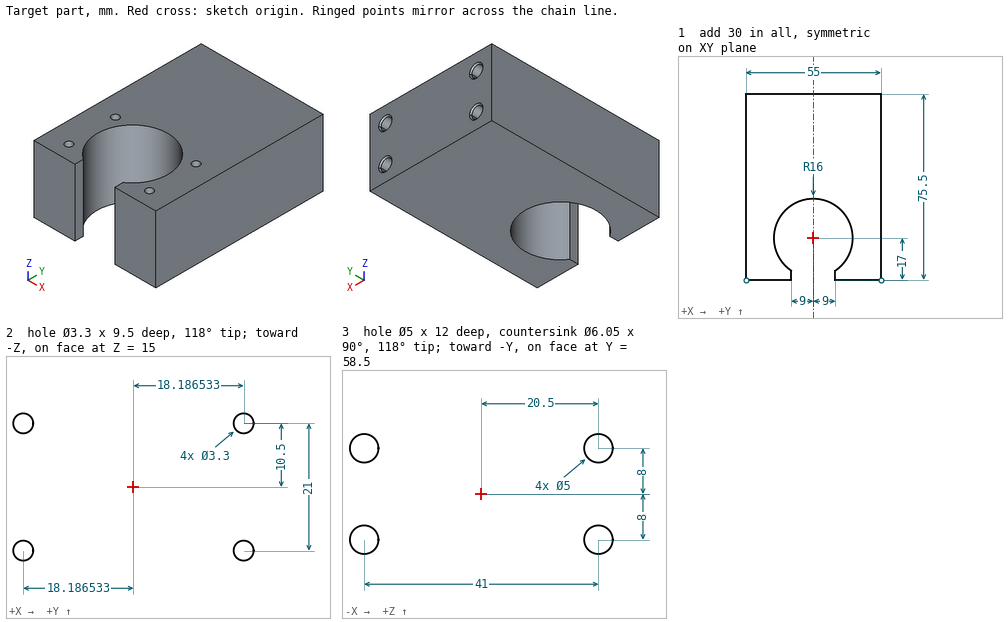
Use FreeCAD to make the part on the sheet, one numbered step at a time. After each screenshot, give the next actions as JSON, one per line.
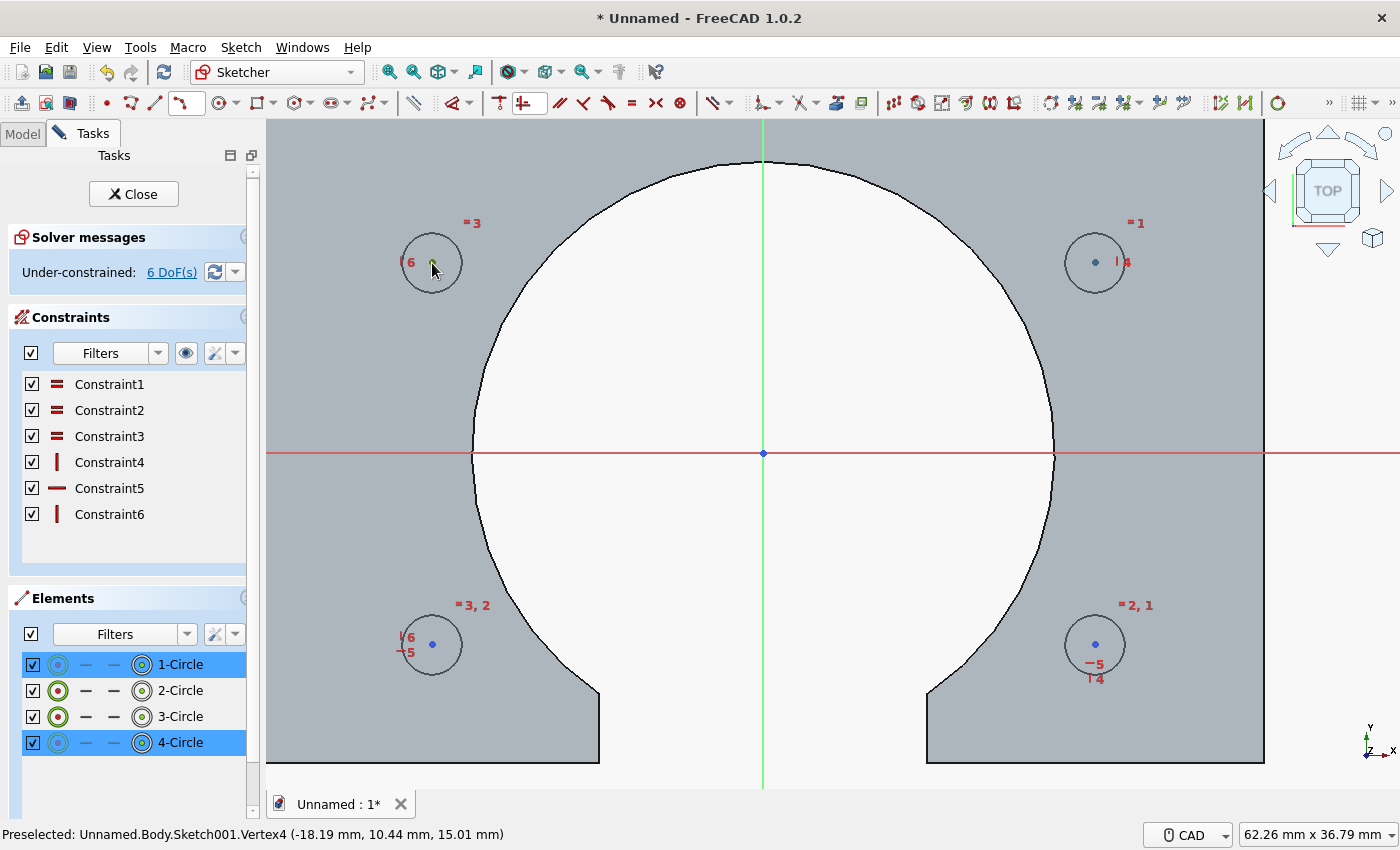
{"action": "left_click", "coordinate": [542, 104]}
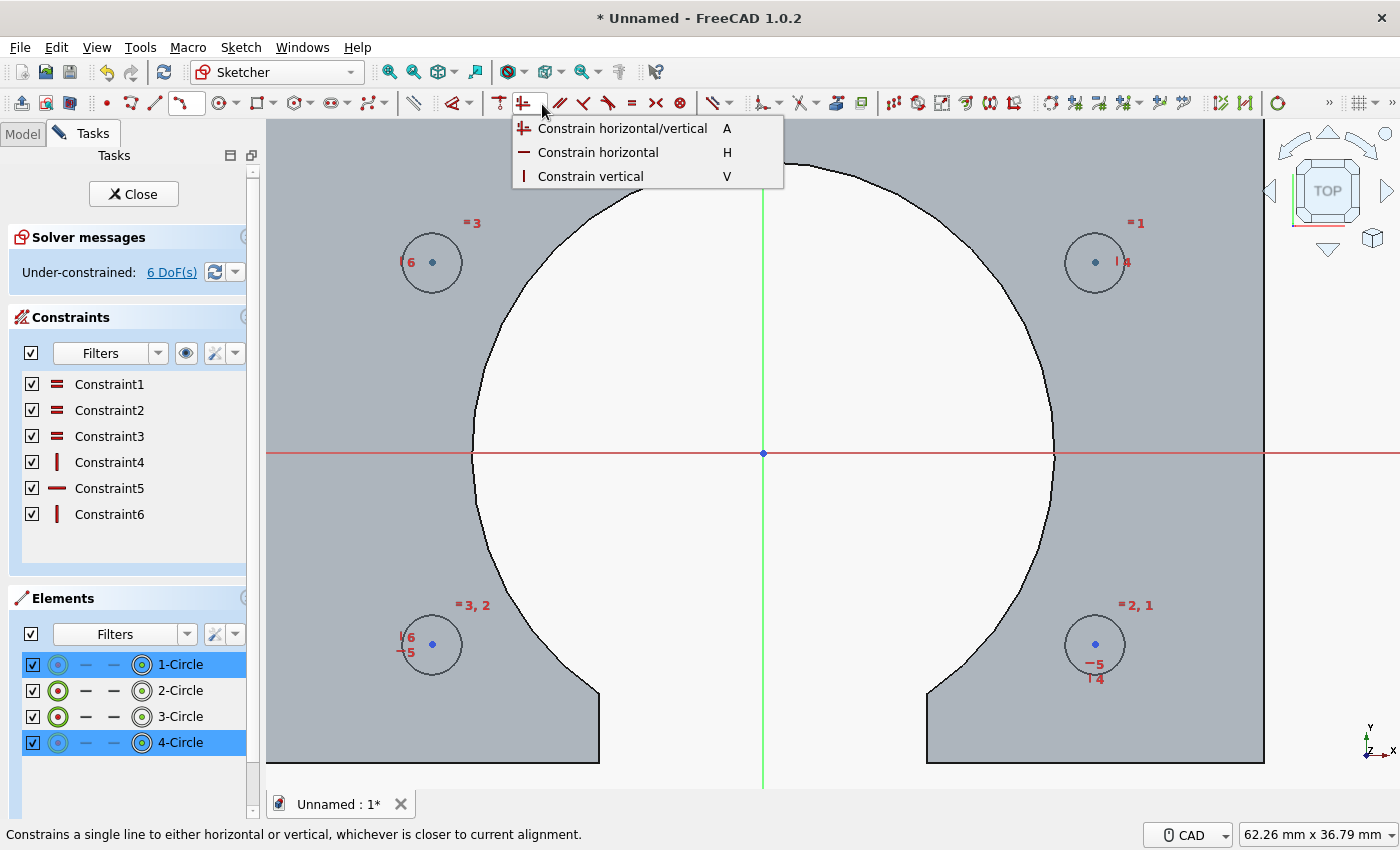
{"action": "left_click", "coordinate": [648, 152]}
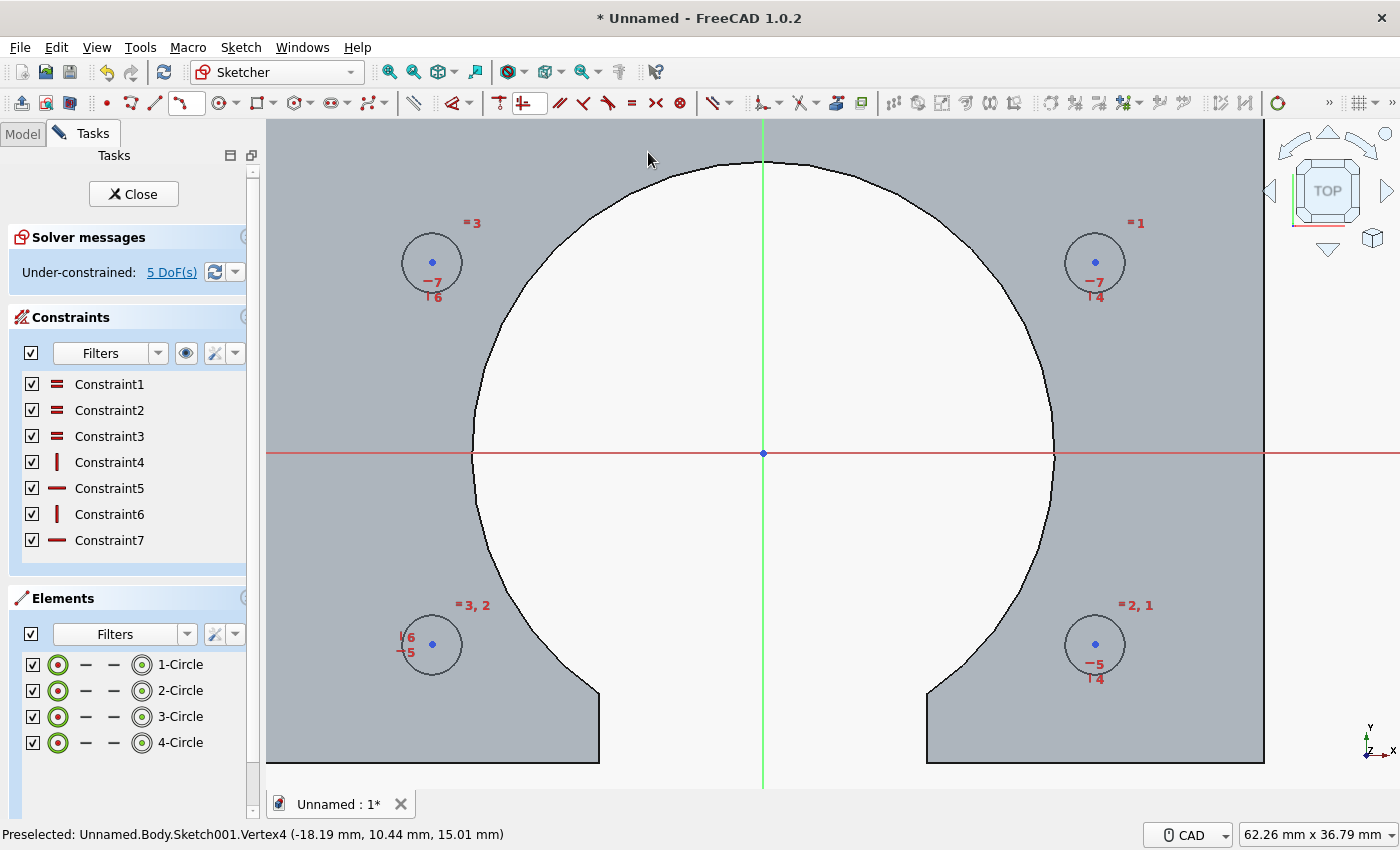
{"action": "left_click", "coordinate": [452, 104]}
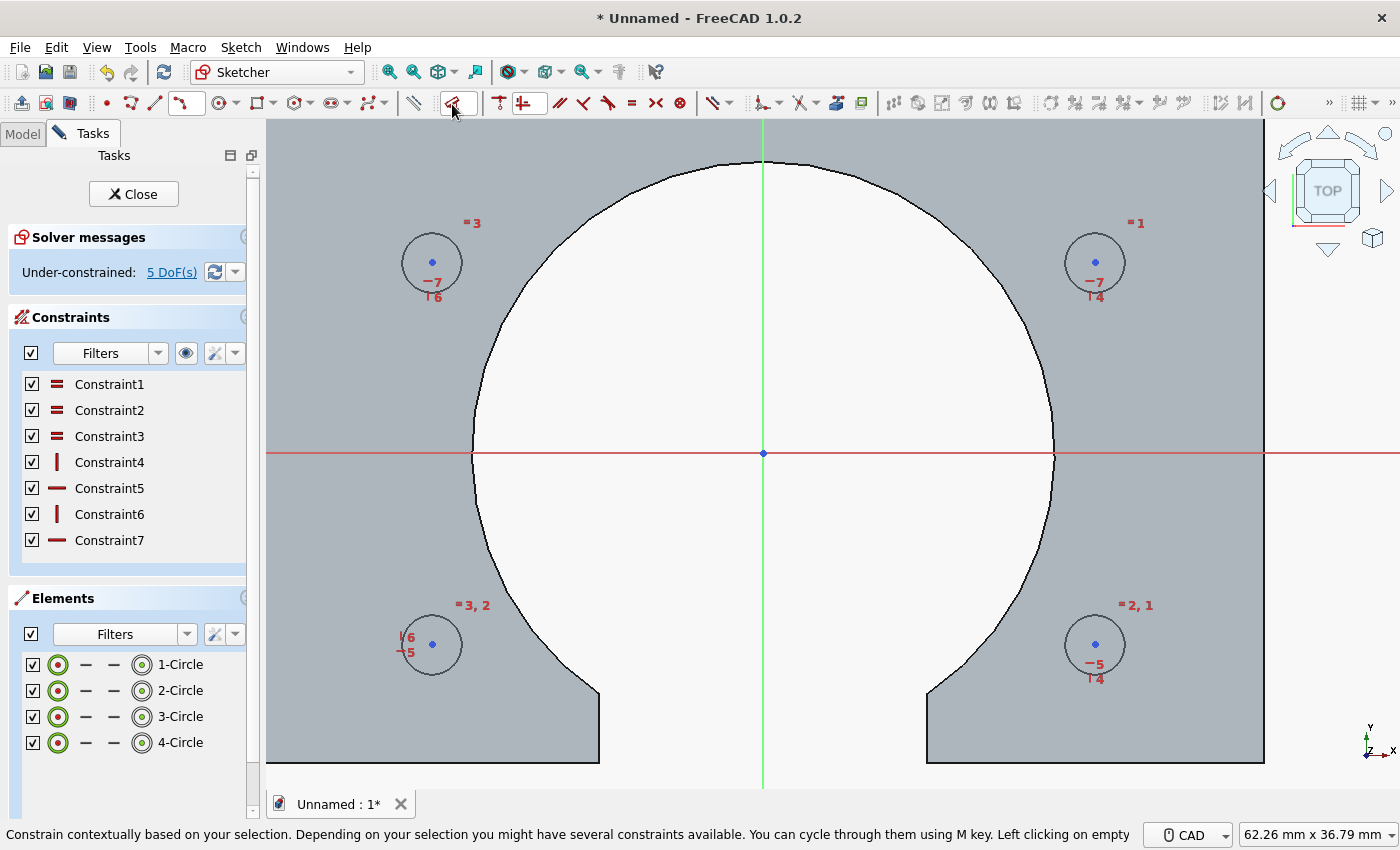
{"action": "left_click", "coordinate": [1116, 242]}
{"action": "left_click", "coordinate": [1139, 219]}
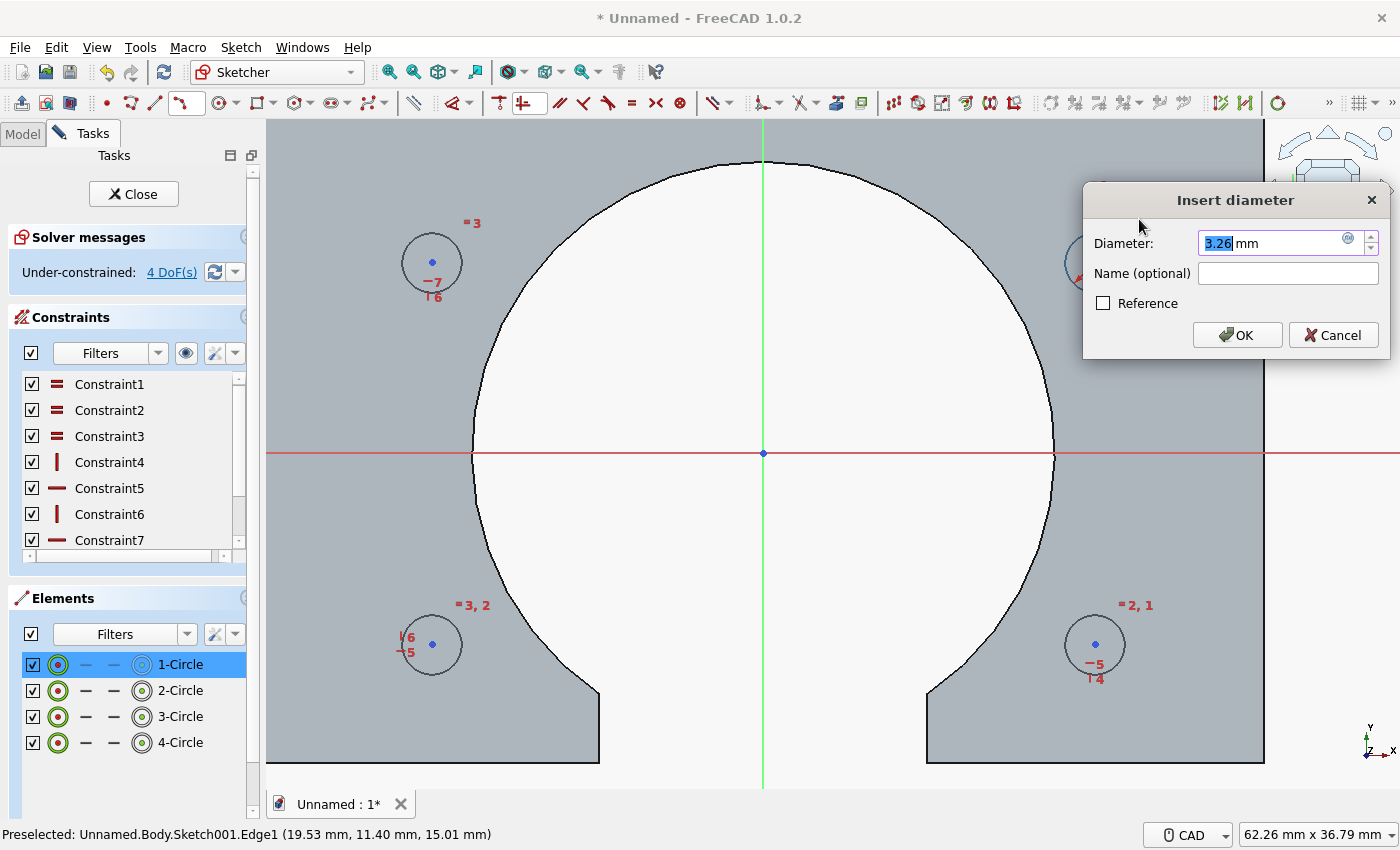
{"action": "type", "text": "3.3"}
{"action": "key", "text": "Return"}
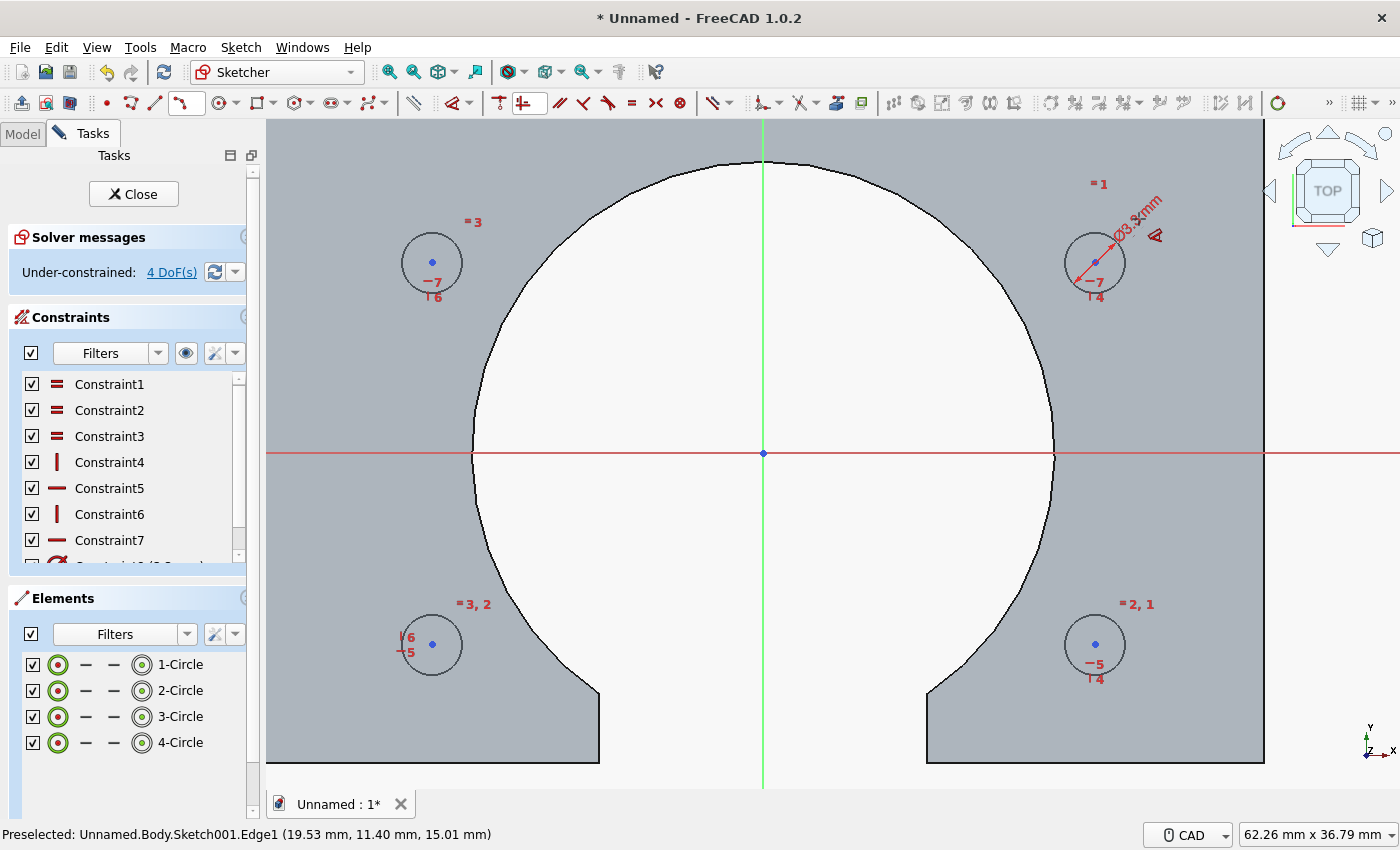
{"action": "left_click", "coordinate": [1095, 263]}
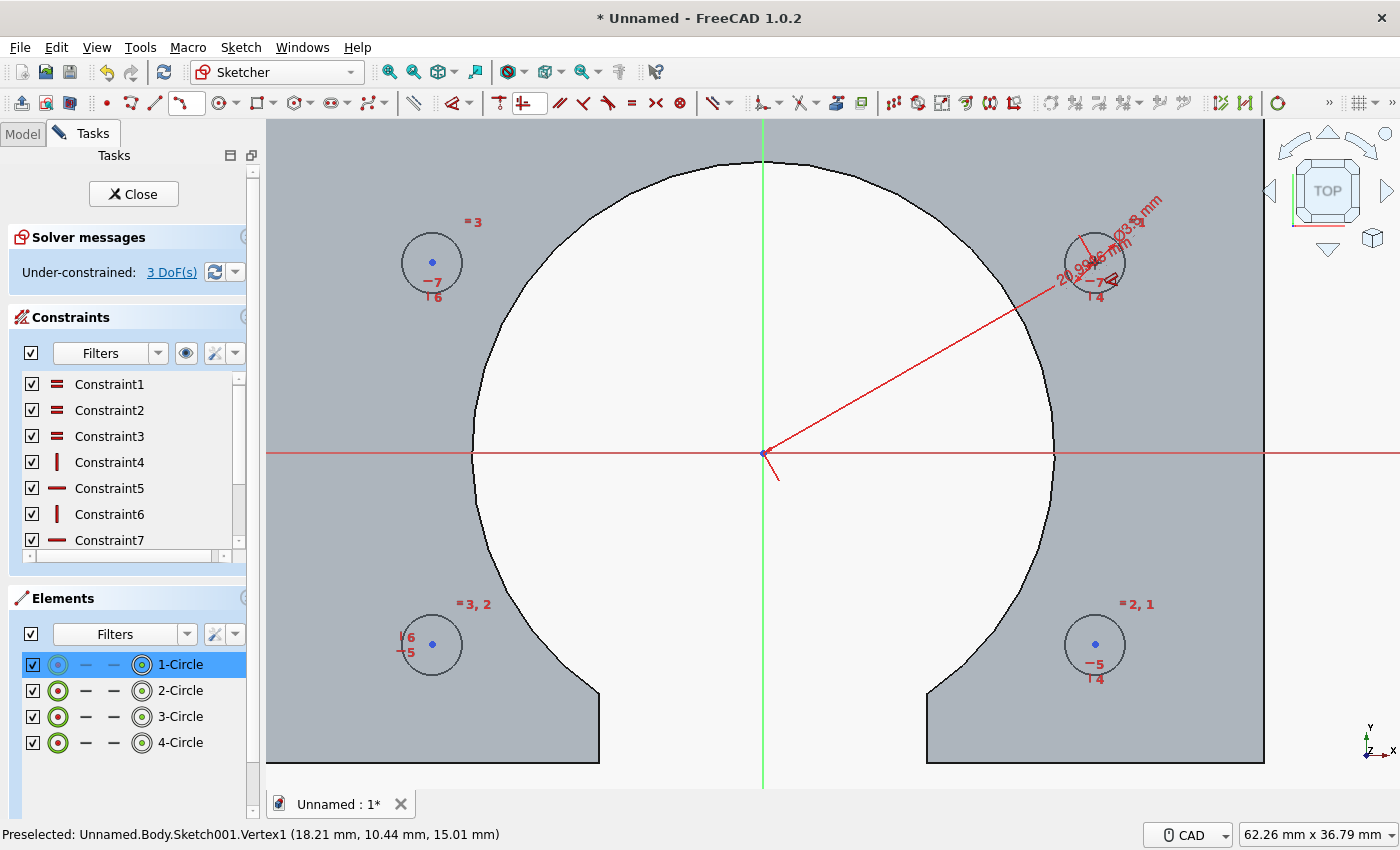
{"action": "left_click", "coordinate": [1095, 645]}
{"action": "left_click", "coordinate": [1129, 366]}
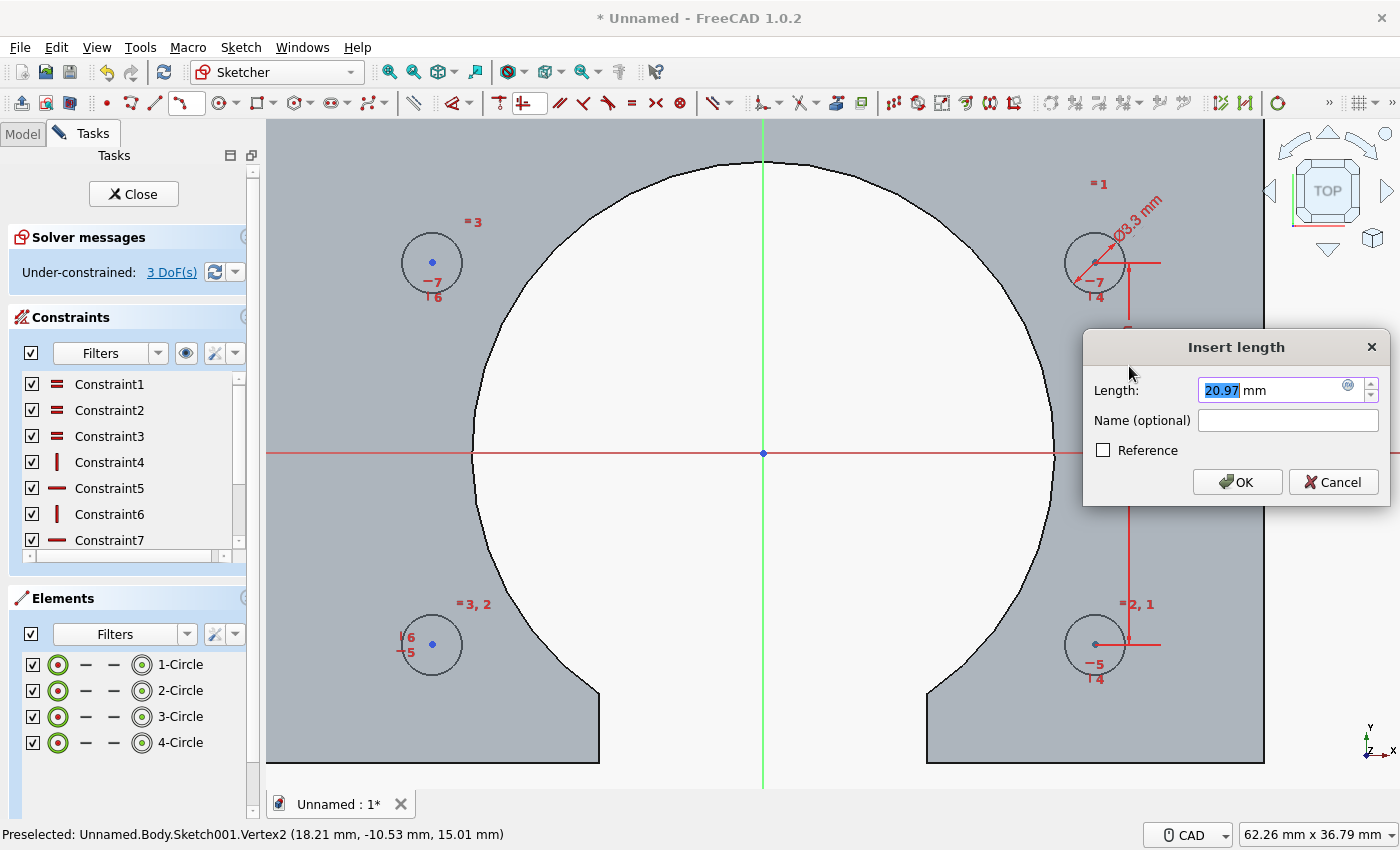
{"action": "type", "text": "21"}
{"action": "key", "text": "Return"}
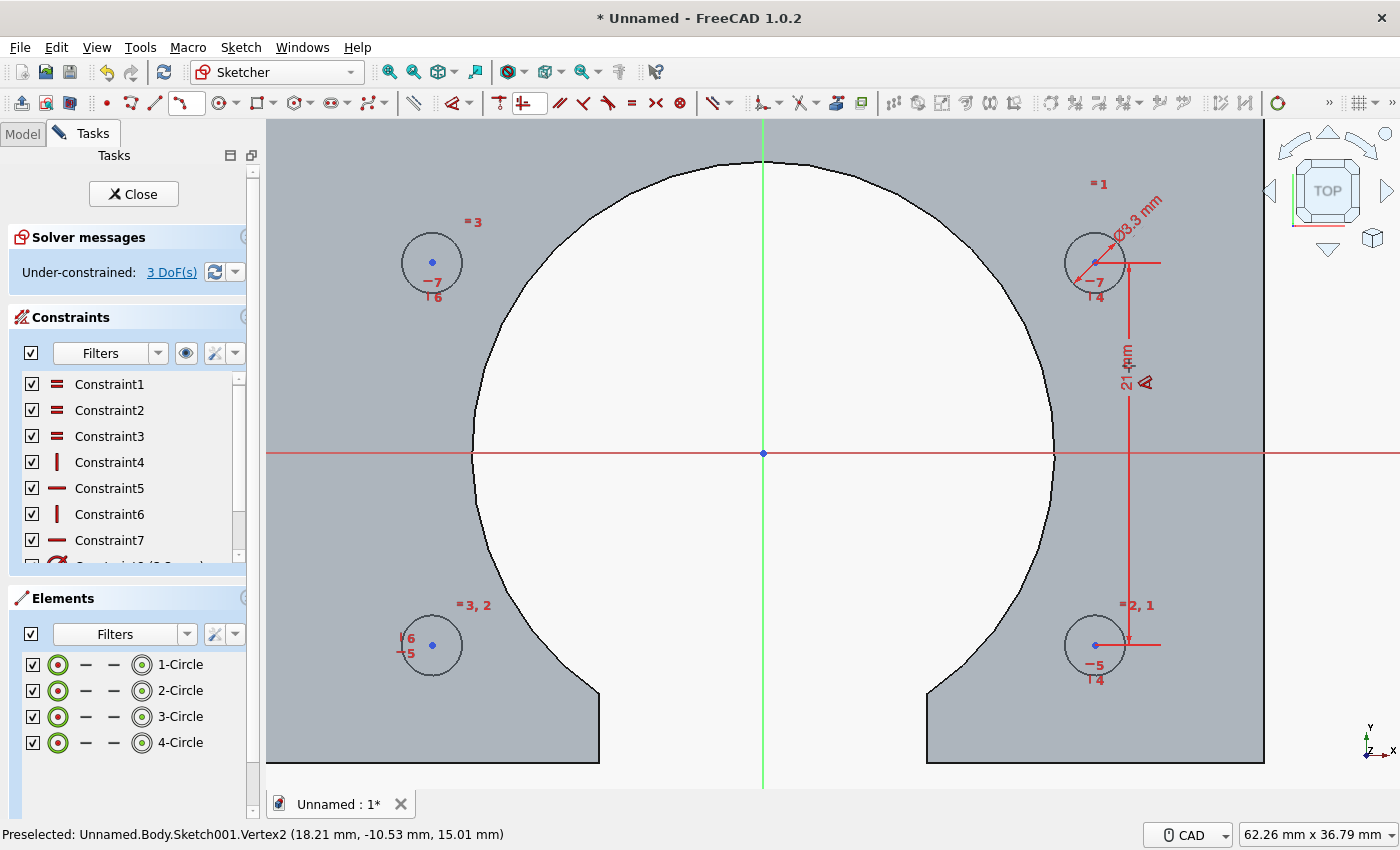
{"action": "left_click", "coordinate": [1095, 263]}
{"action": "left_click", "coordinate": [1129, 314]}